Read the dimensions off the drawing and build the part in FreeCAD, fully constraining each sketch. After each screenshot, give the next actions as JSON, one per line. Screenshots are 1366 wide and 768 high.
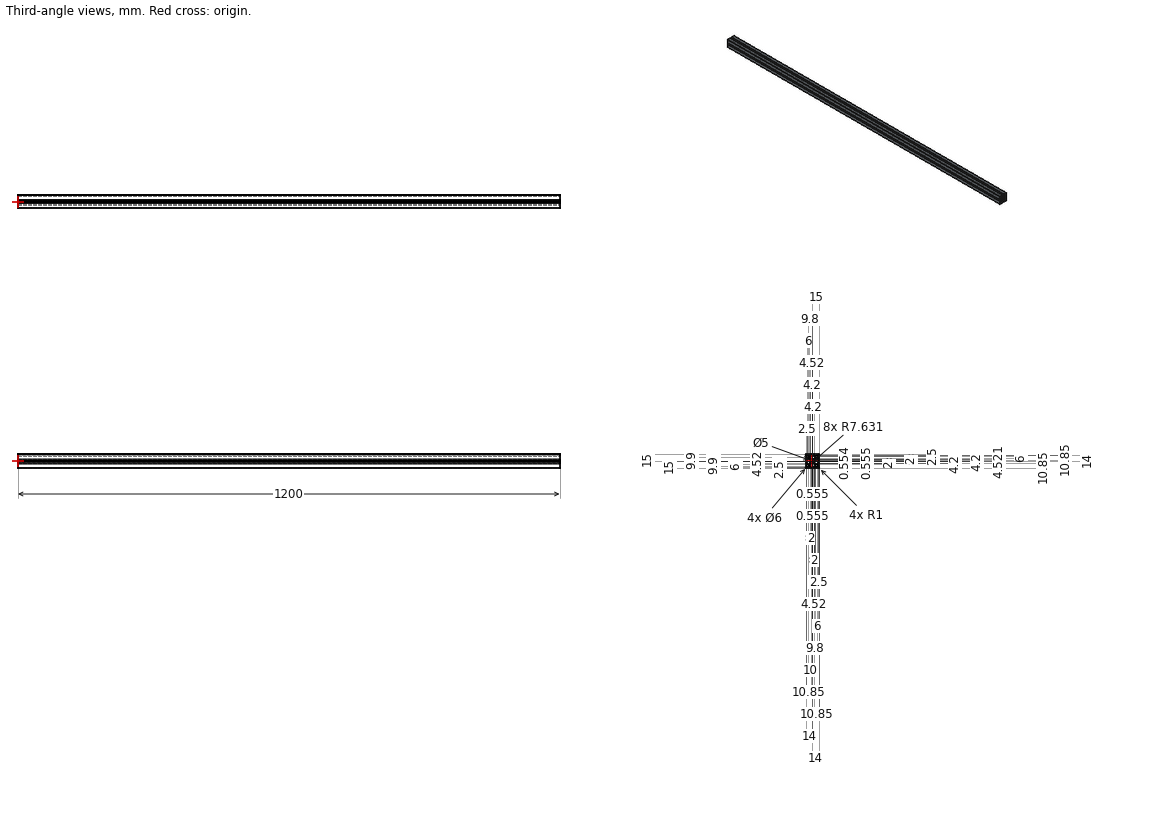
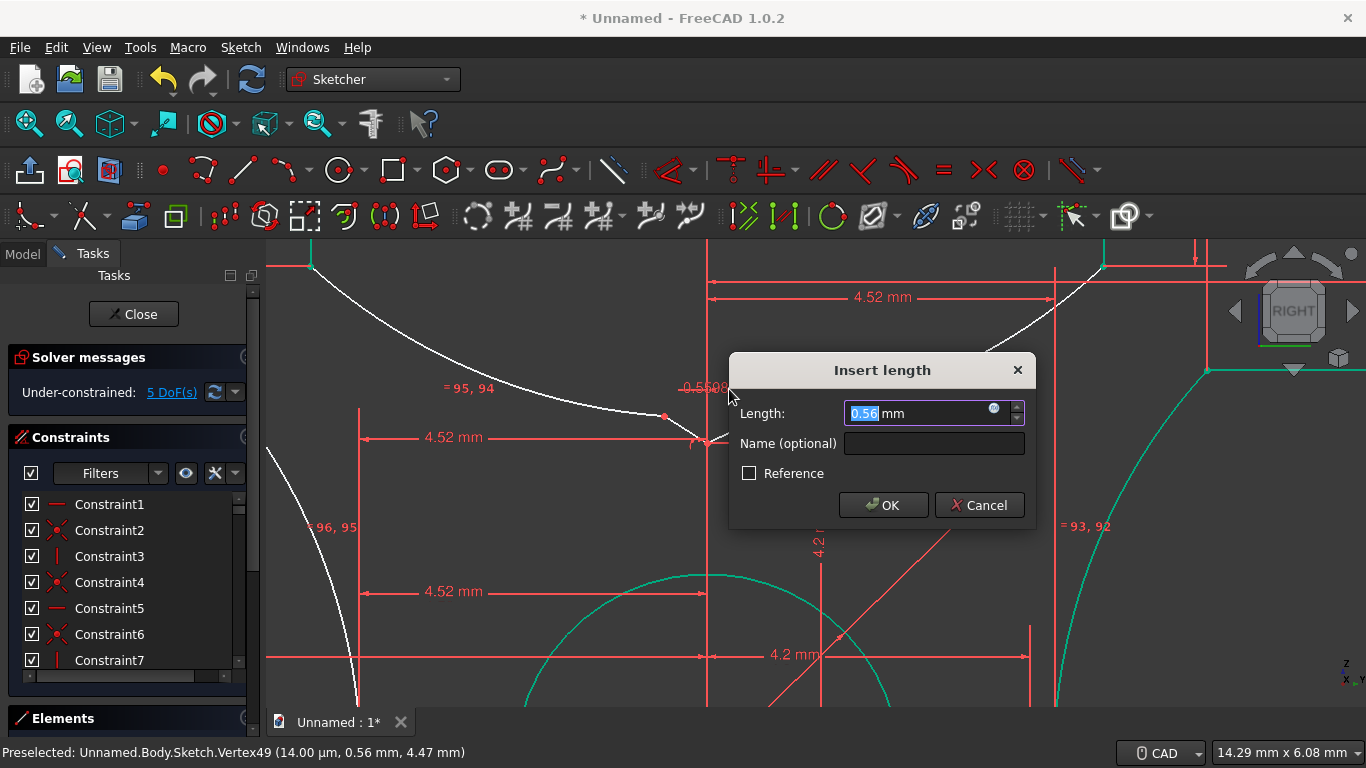
{"action": "type", "text": "0.555"}
{"action": "key", "text": "Return"}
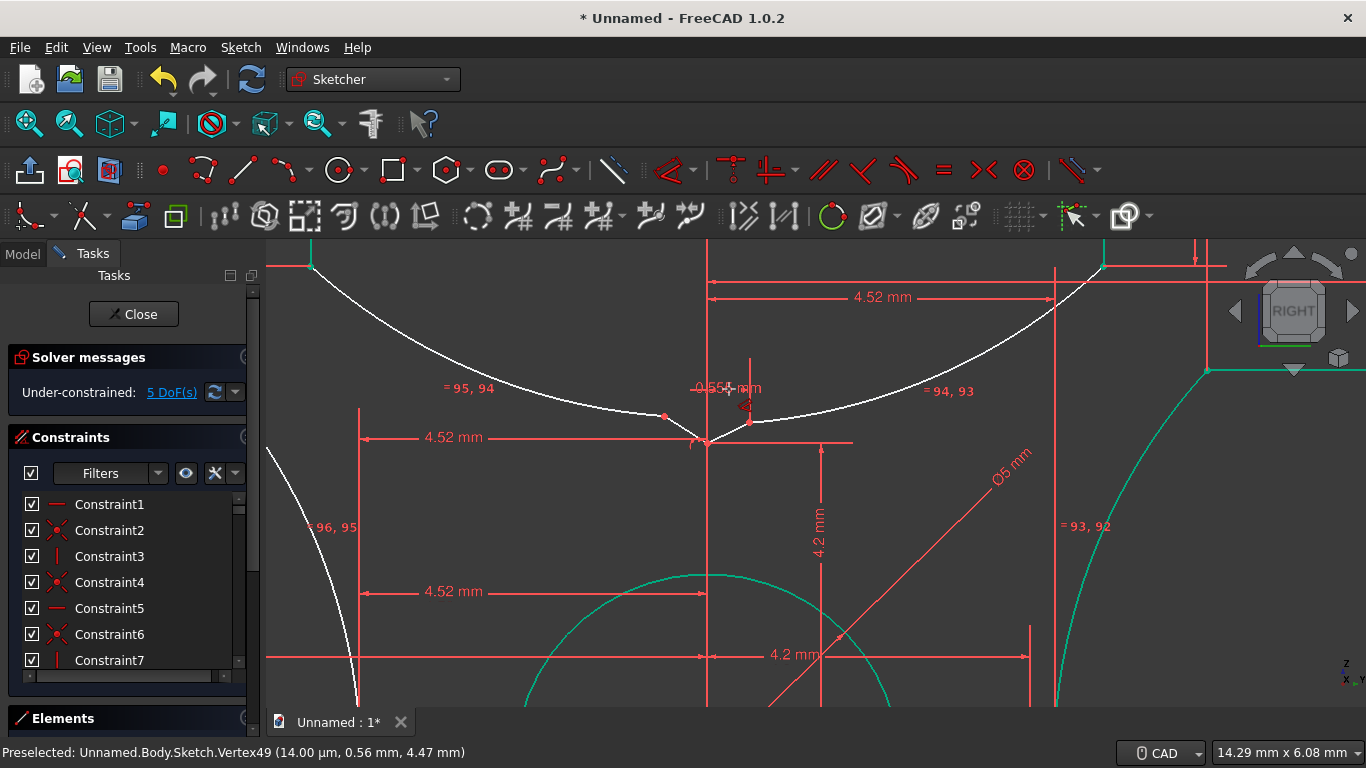
{"action": "scroll", "coordinate": [754, 427], "scroll_direction": "down", "scroll_amount": 10}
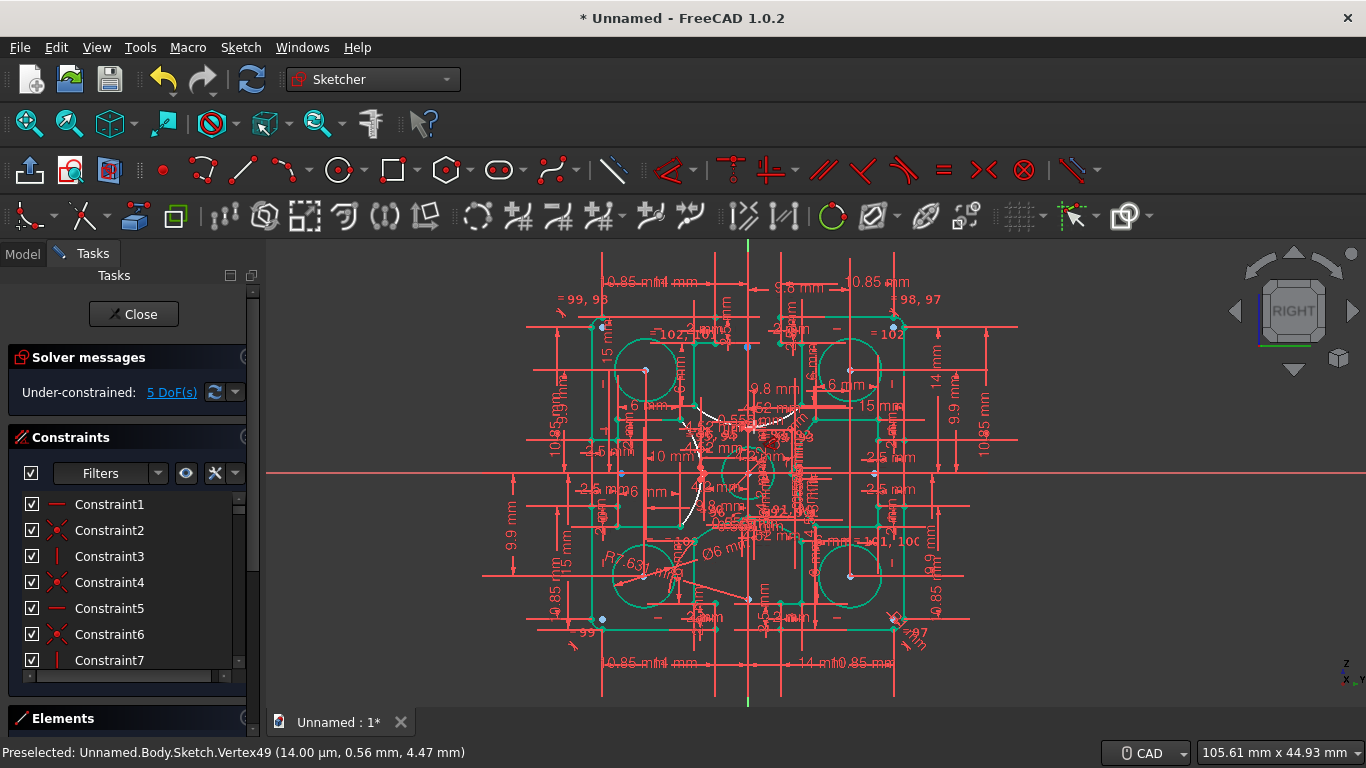
{"action": "scroll", "coordinate": [754, 427], "scroll_direction": "up", "scroll_amount": 4}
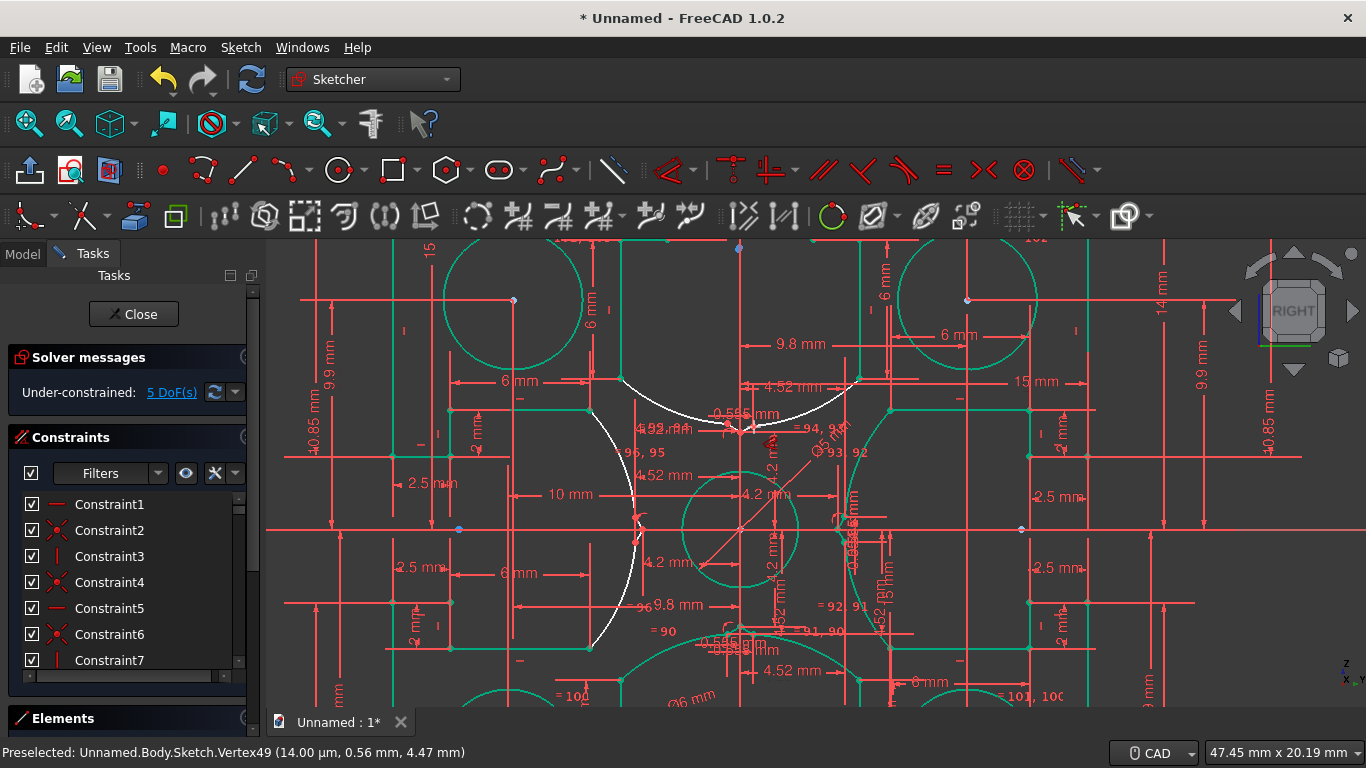
{"action": "left_click", "coordinate": [753, 426]}
{"action": "left_click", "coordinate": [682, 454]}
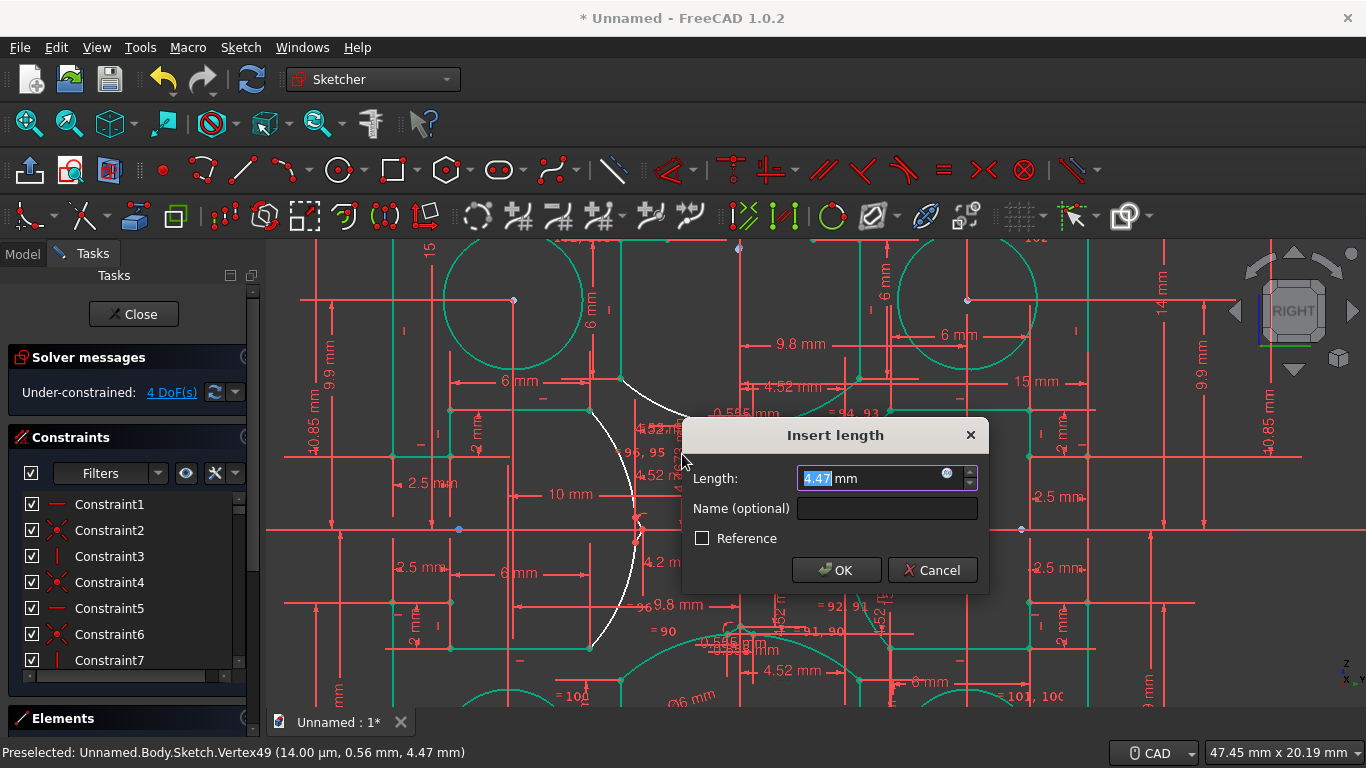
{"action": "type", "text": "4.521"}
{"action": "key", "text": "Return"}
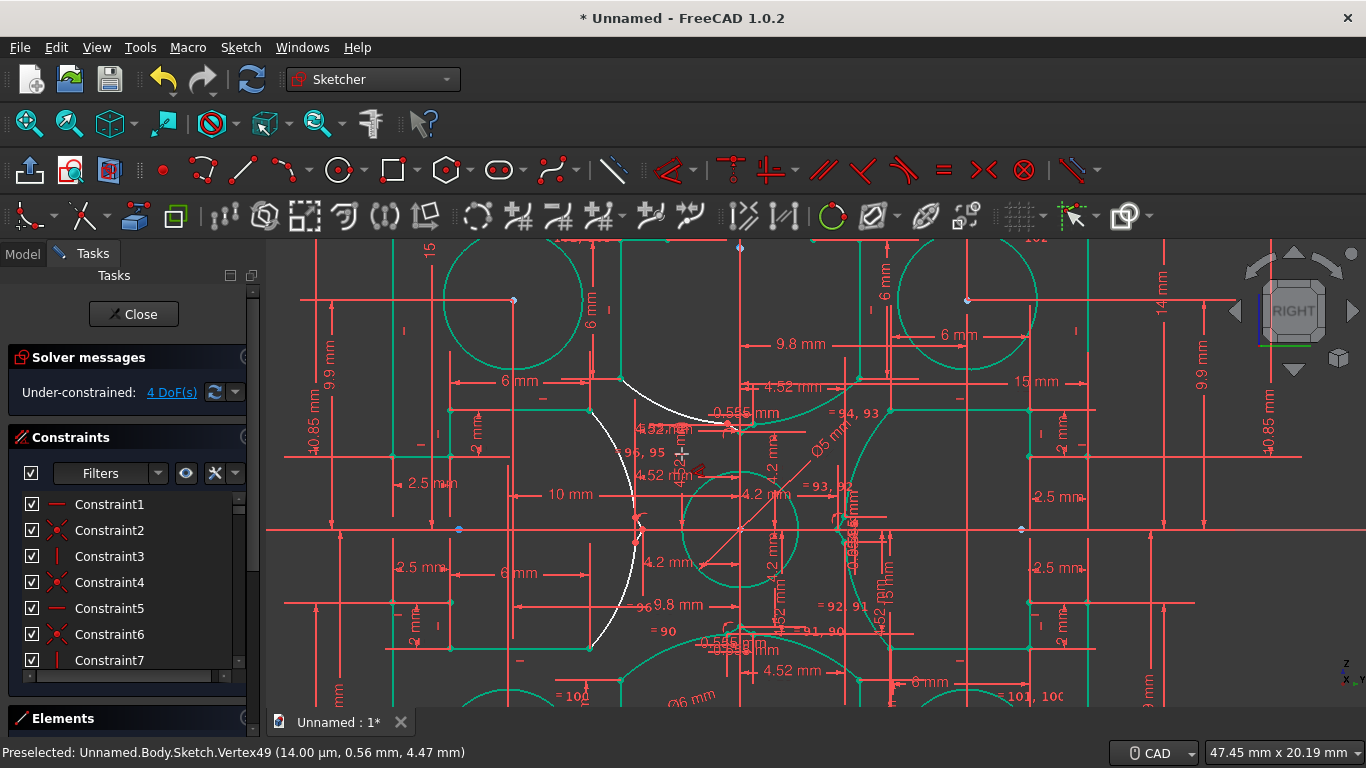
{"action": "scroll", "coordinate": [727, 424], "scroll_direction": "up", "scroll_amount": 6}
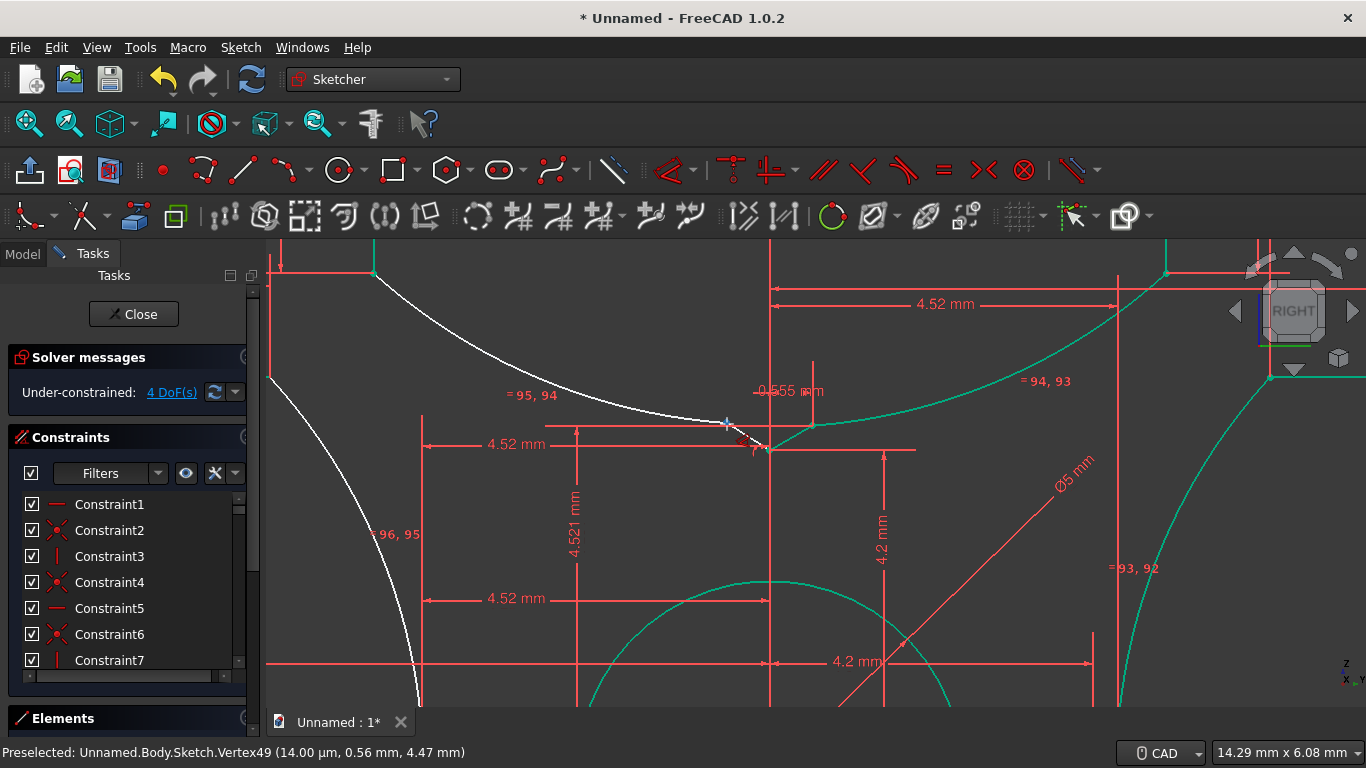
{"action": "left_click", "coordinate": [727, 423]}
{"action": "left_click", "coordinate": [748, 365]}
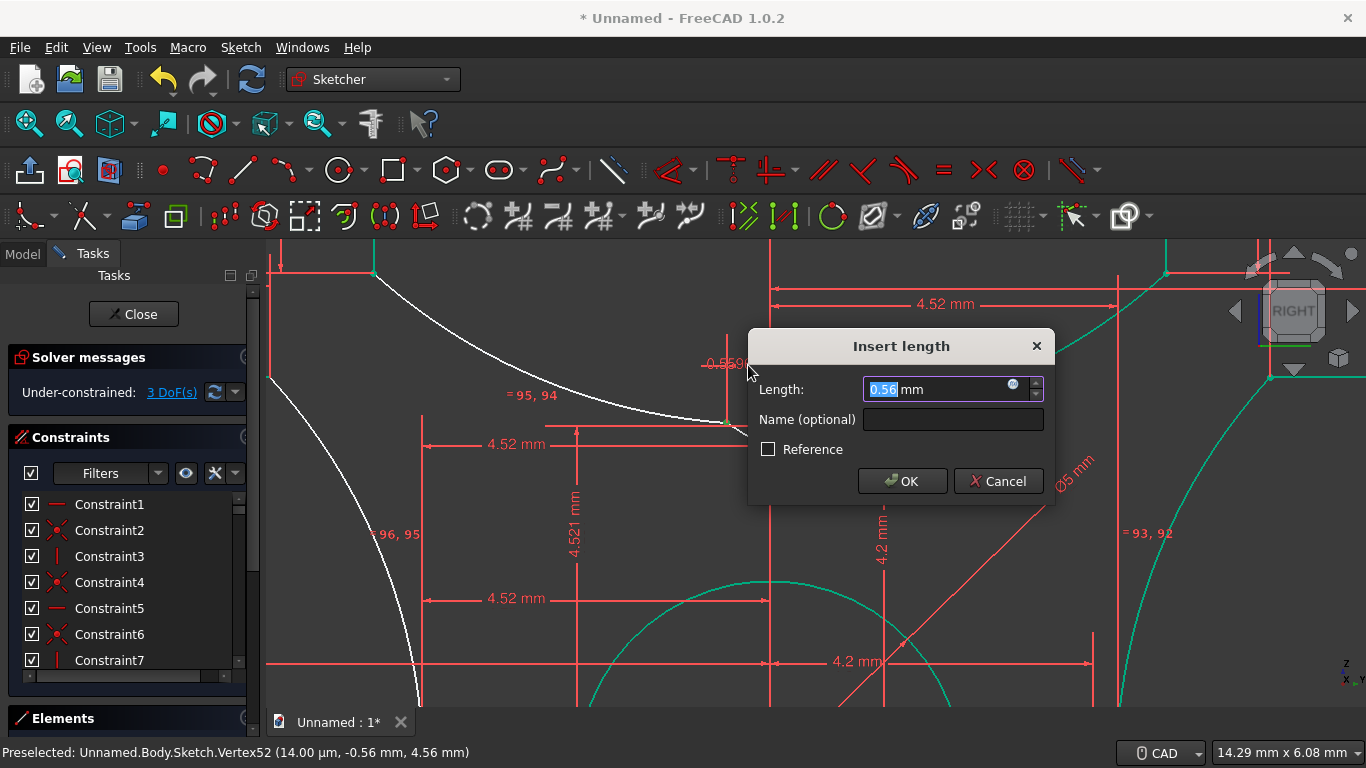
{"action": "type", "text": "0.555"}
{"action": "key", "text": "Return"}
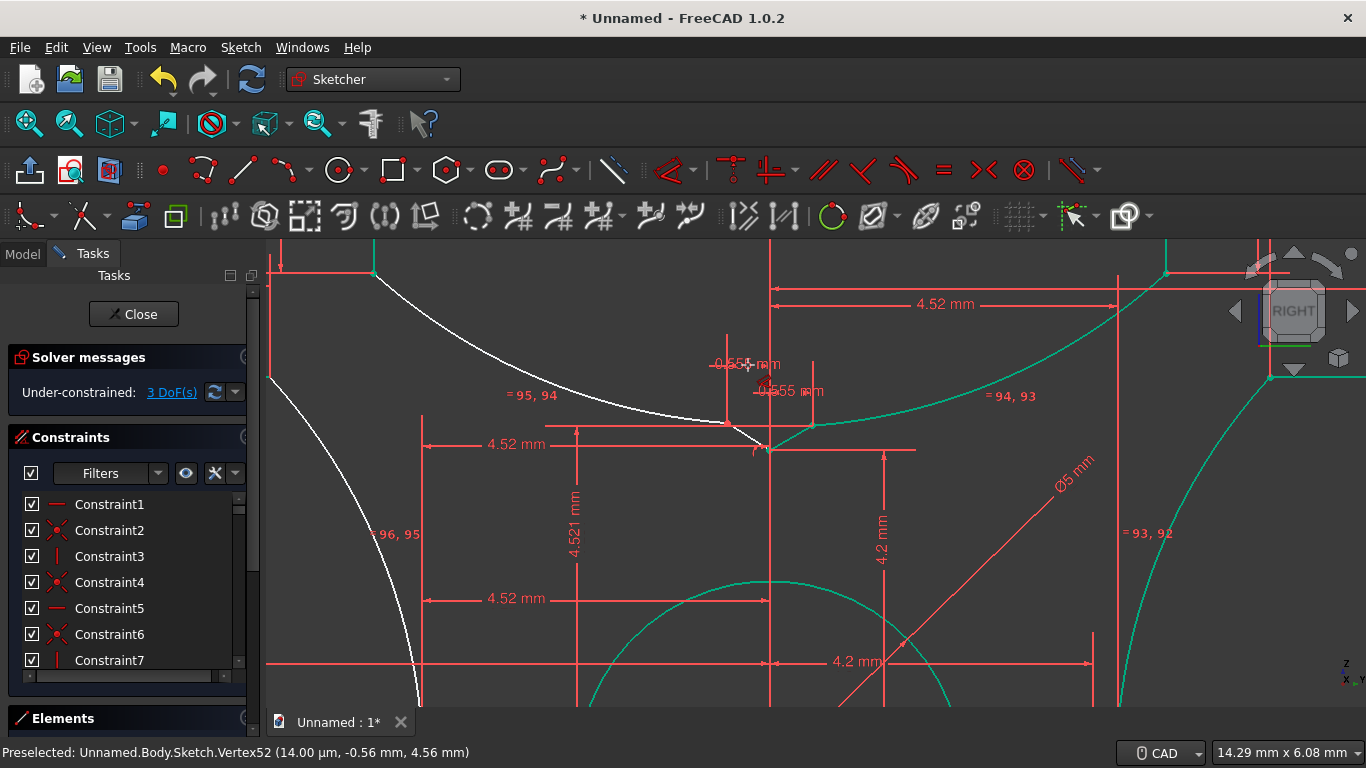
{"action": "scroll", "coordinate": [744, 426], "scroll_direction": "down", "scroll_amount": 10}